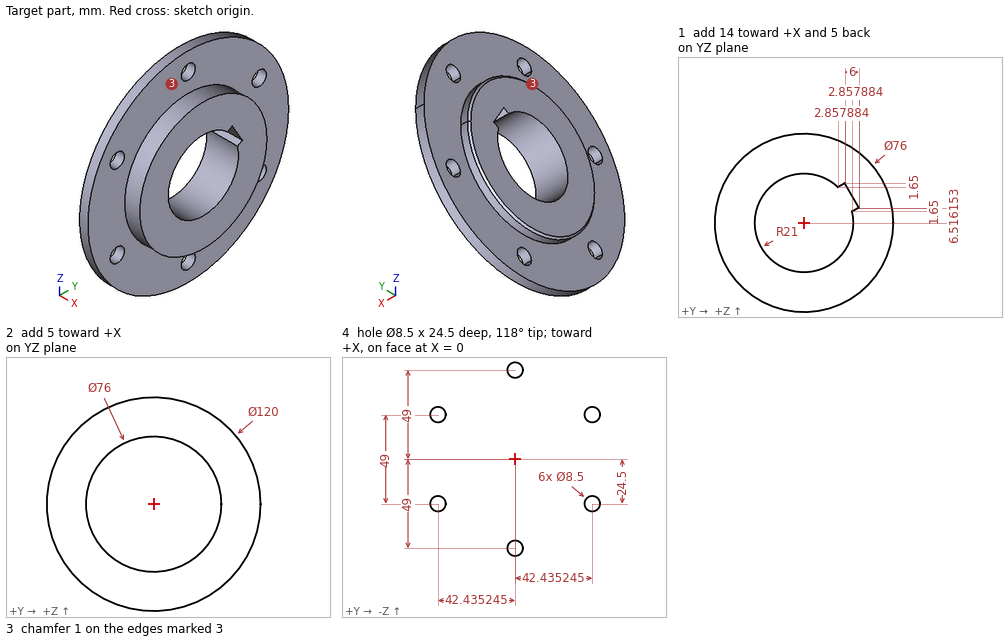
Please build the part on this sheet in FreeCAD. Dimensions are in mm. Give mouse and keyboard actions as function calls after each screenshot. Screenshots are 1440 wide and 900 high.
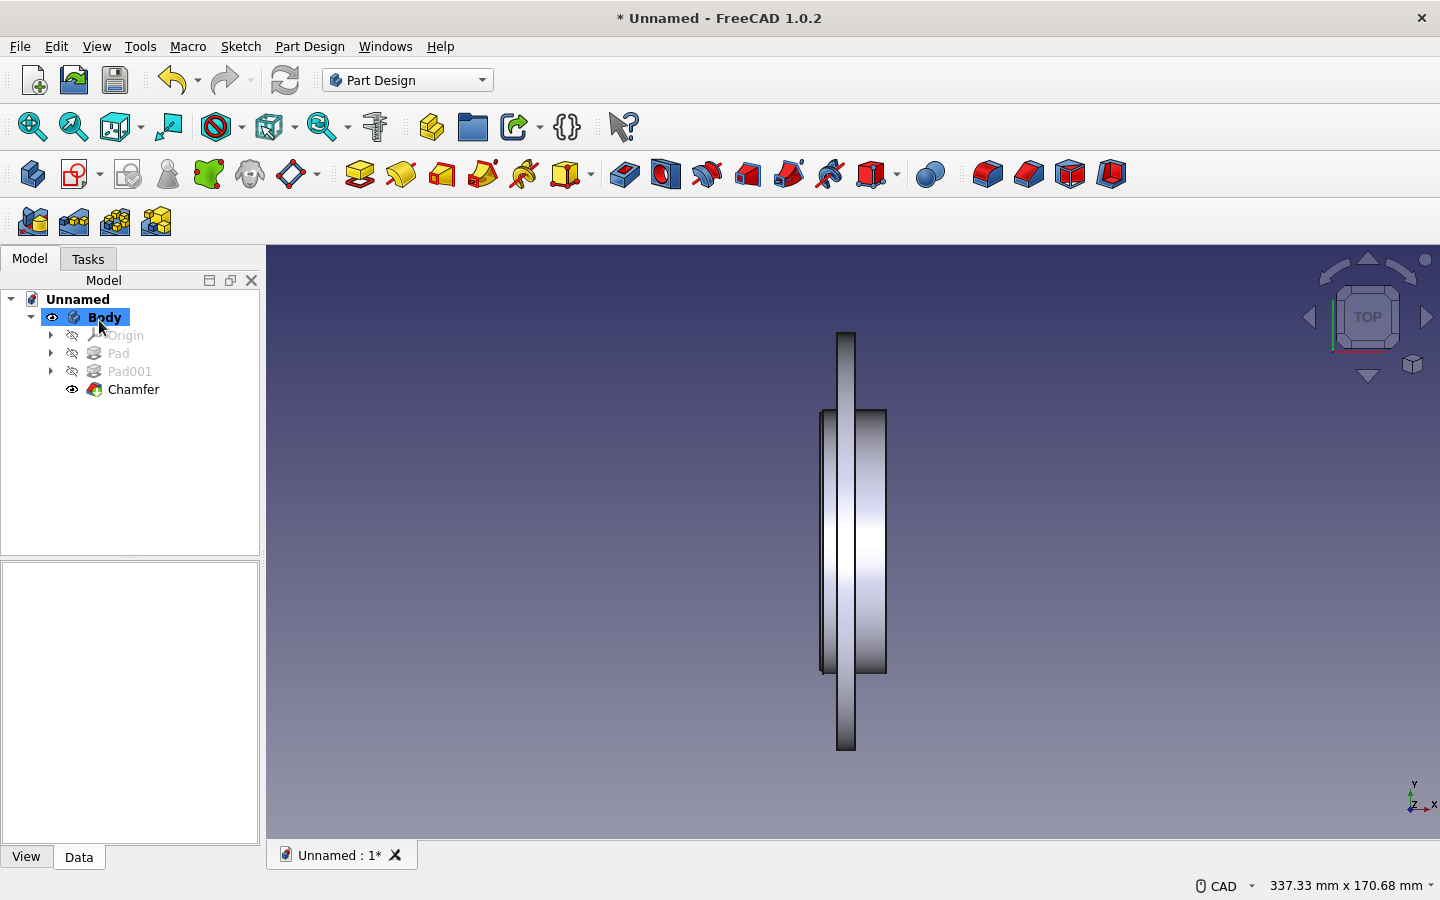
key(6)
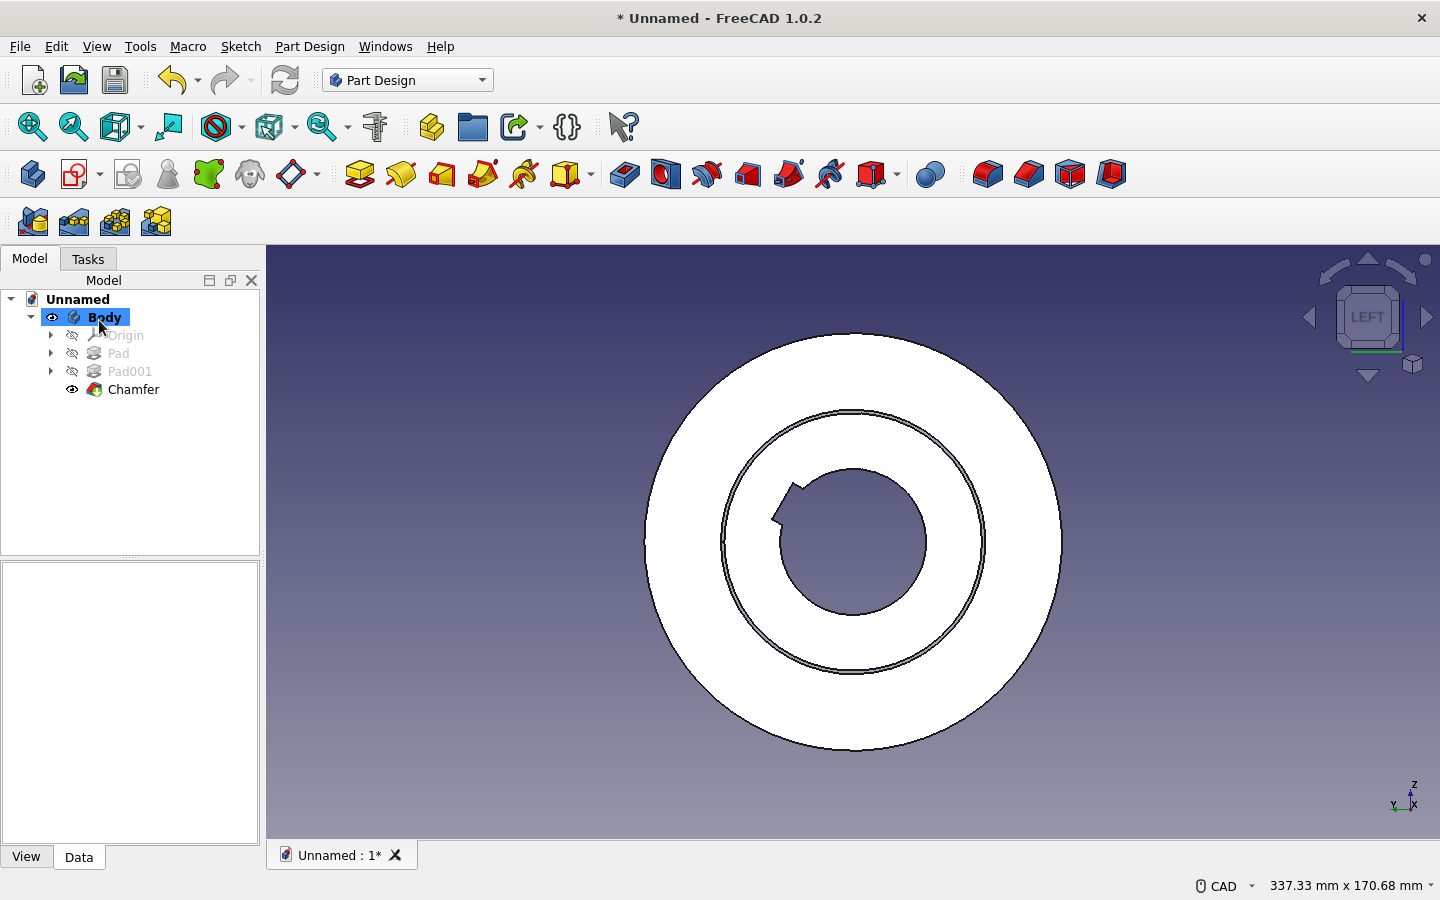
click(972, 422)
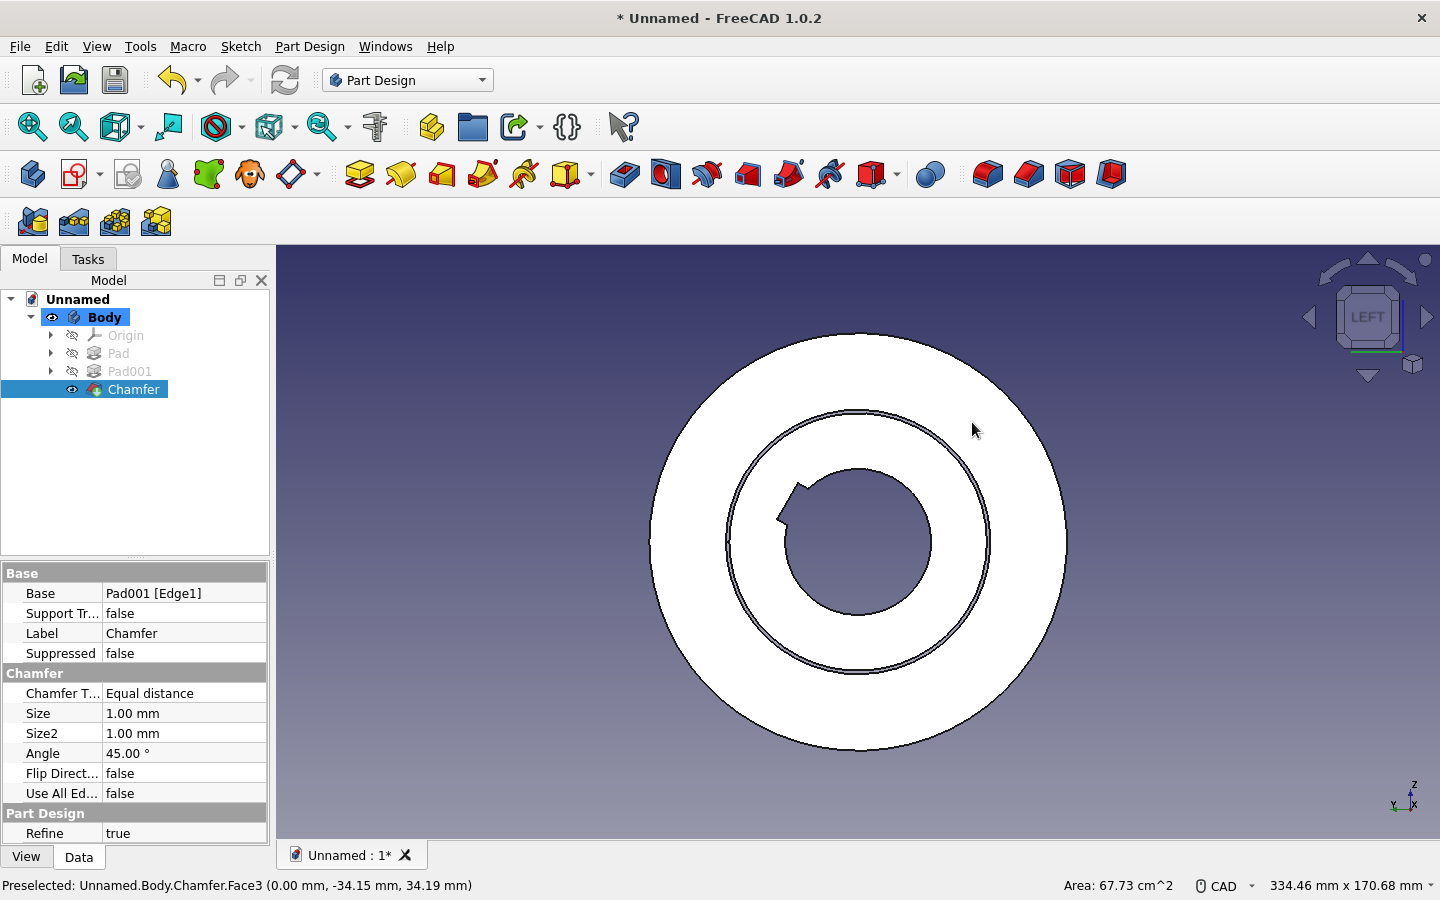
click(74, 174)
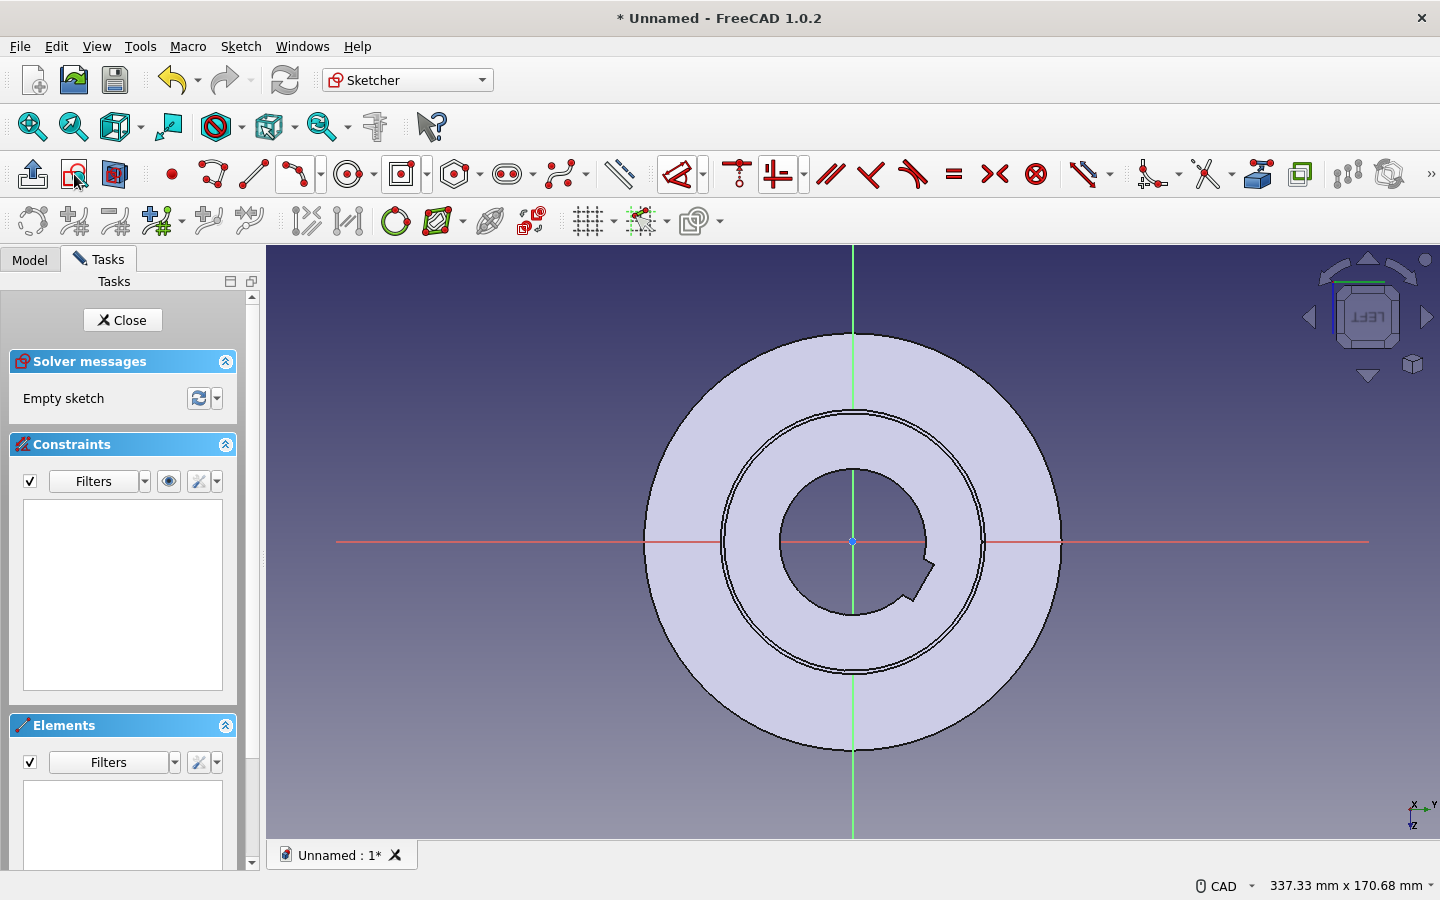
click(115, 174)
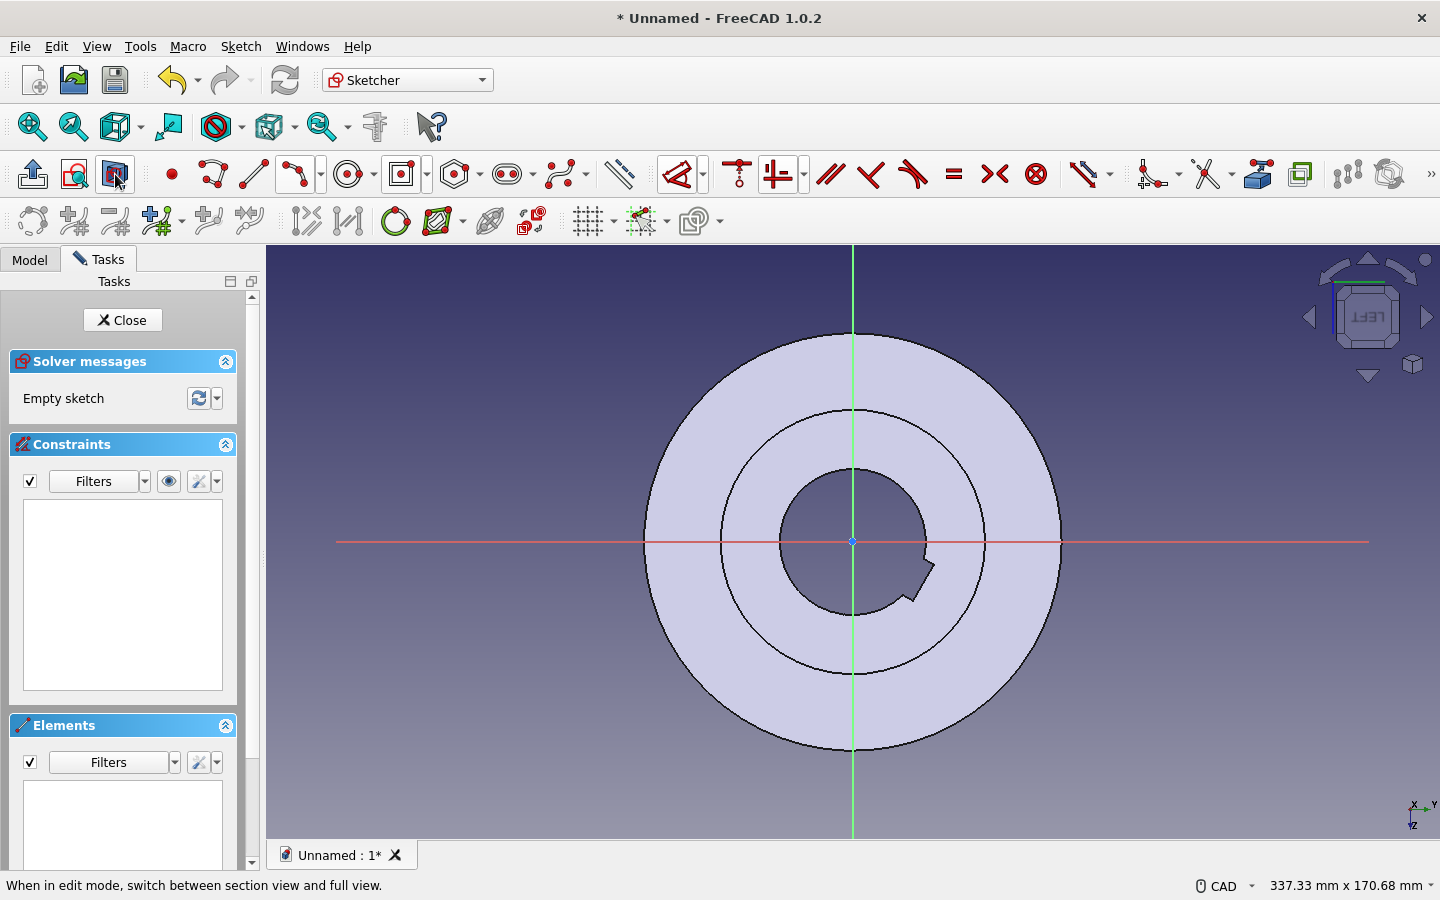
key(g)
key(c)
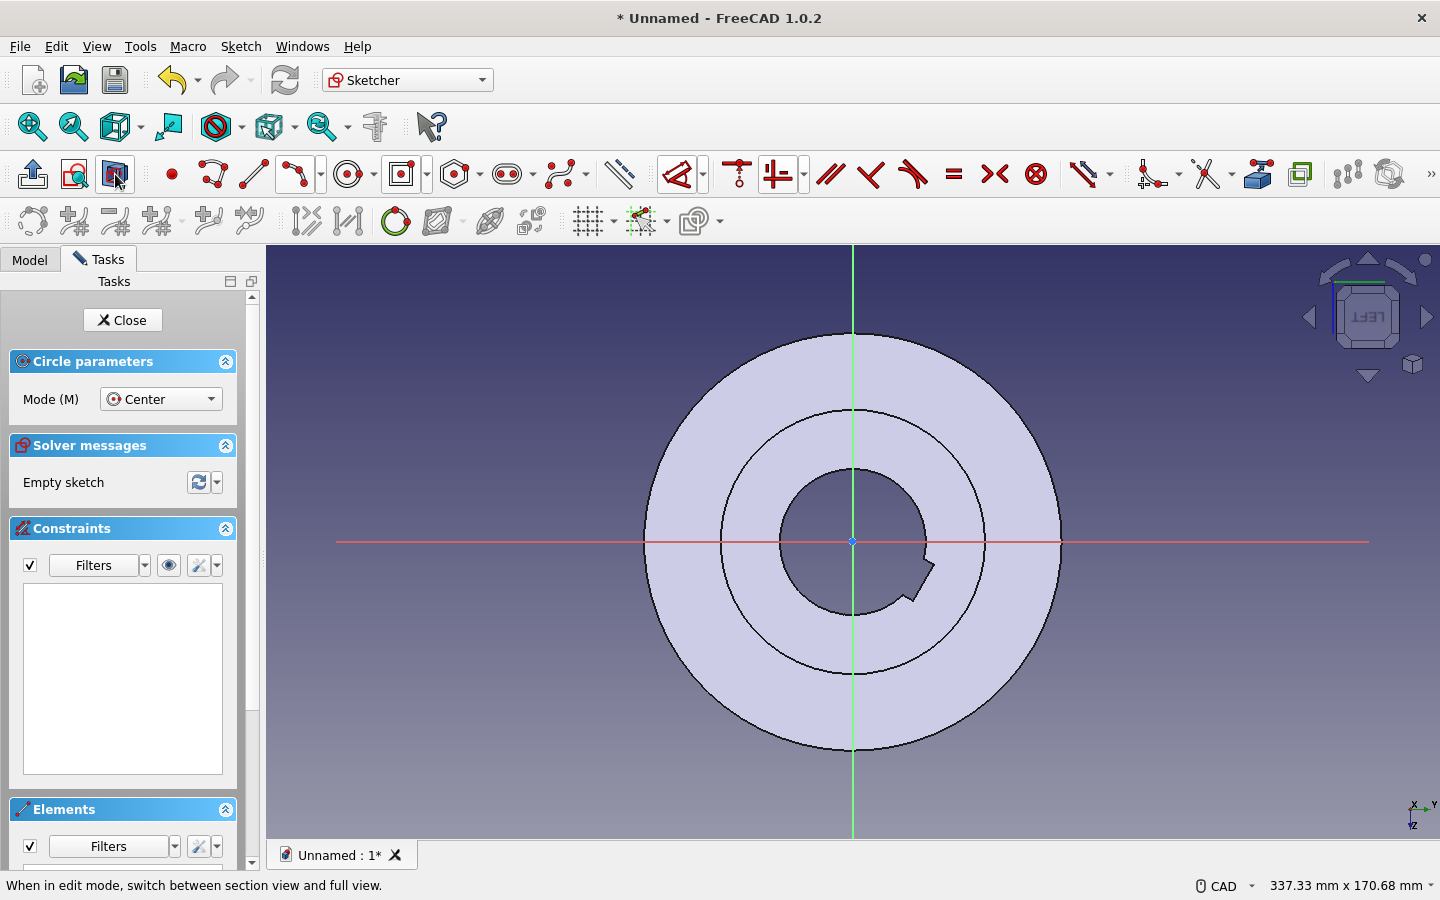
scroll(1001, 627, up, 3)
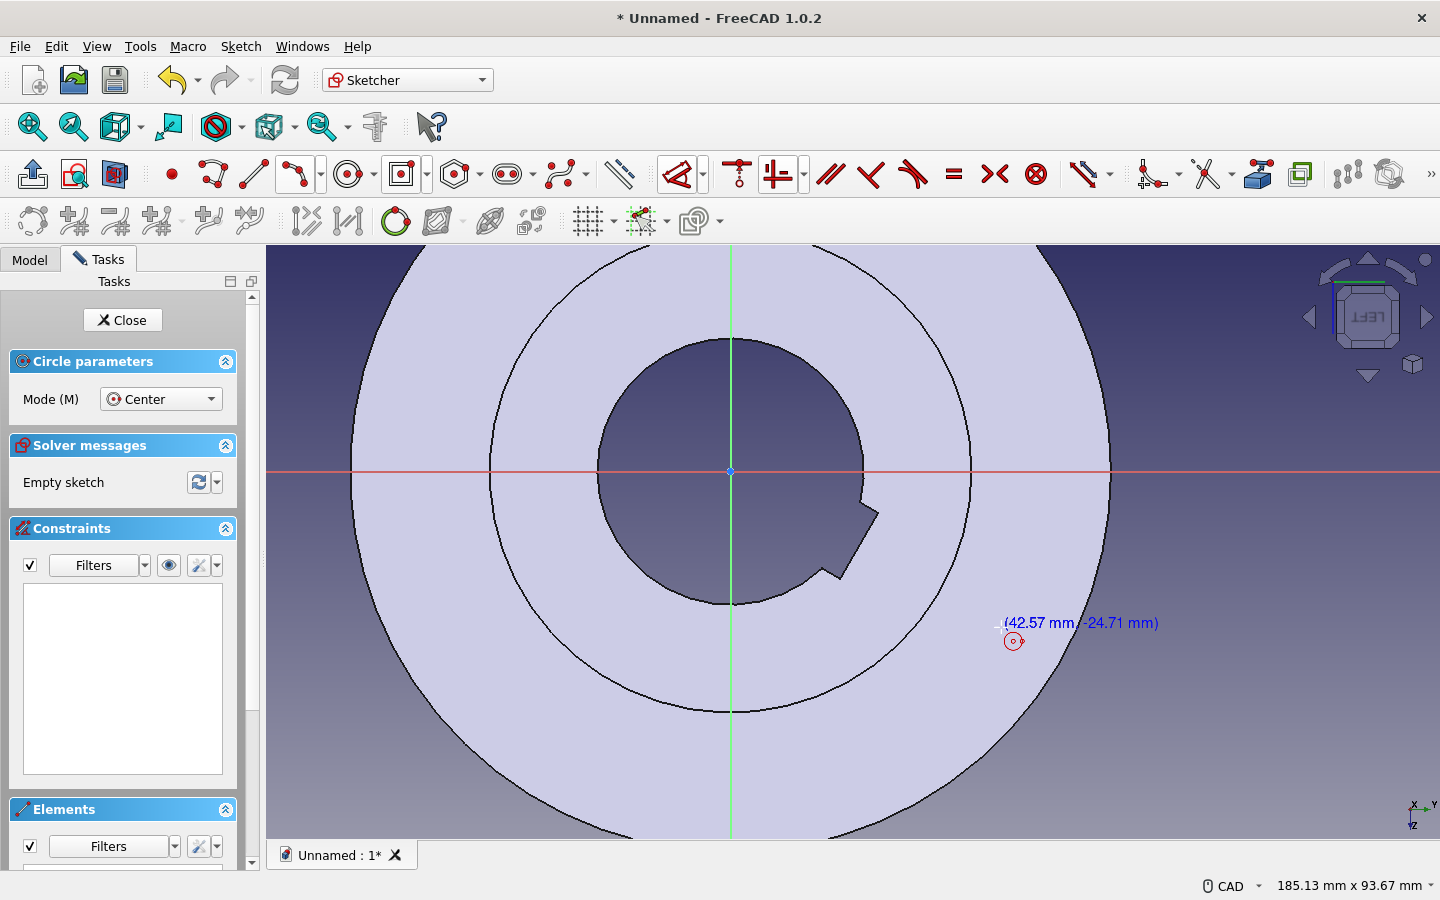
click(1000, 627)
move(1019, 608)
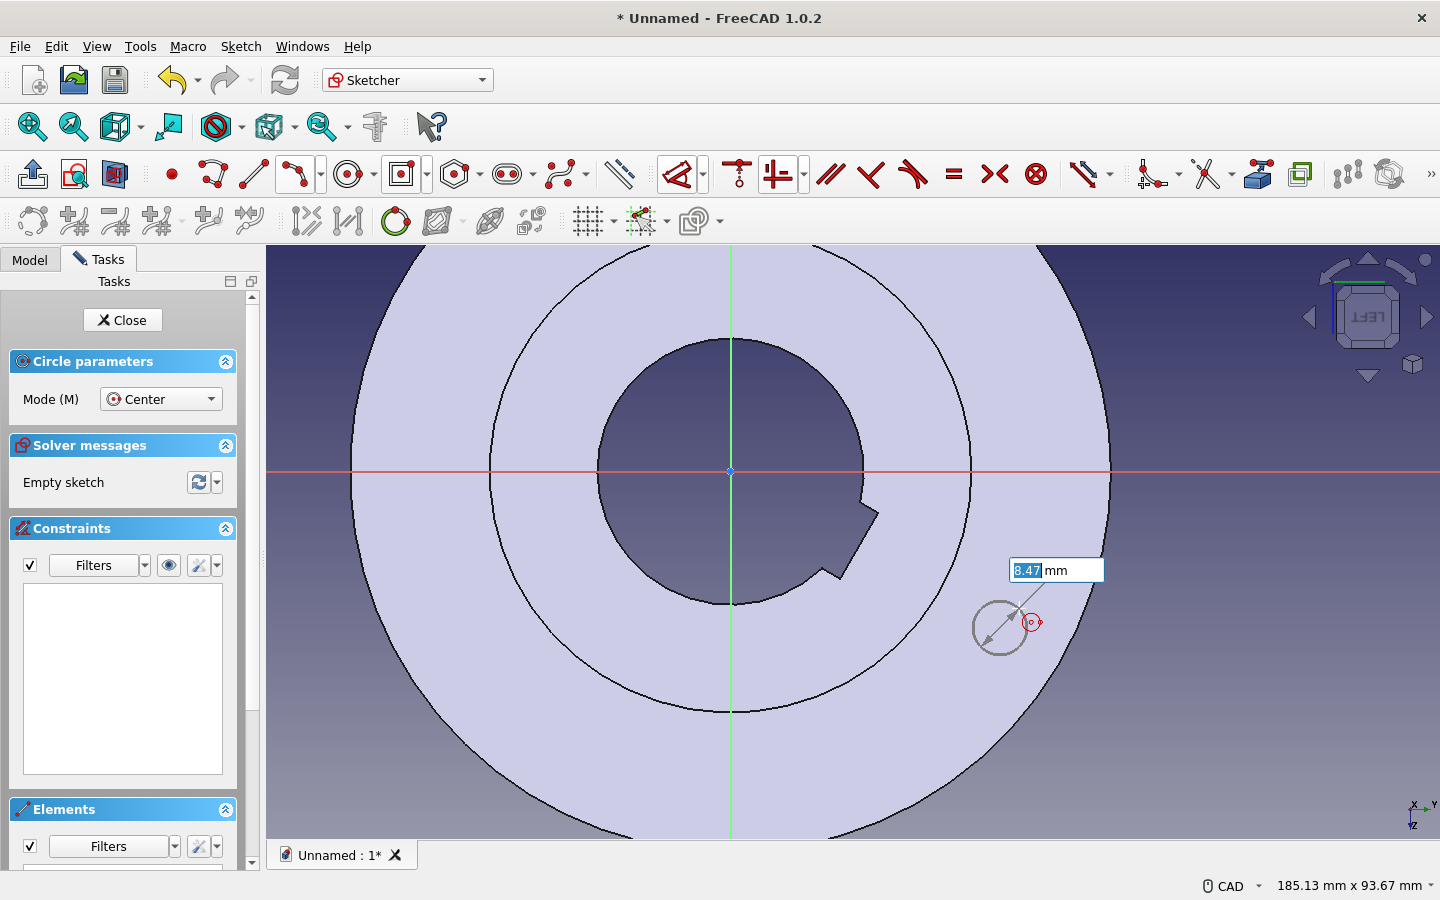
text(8.5)
key(Return)